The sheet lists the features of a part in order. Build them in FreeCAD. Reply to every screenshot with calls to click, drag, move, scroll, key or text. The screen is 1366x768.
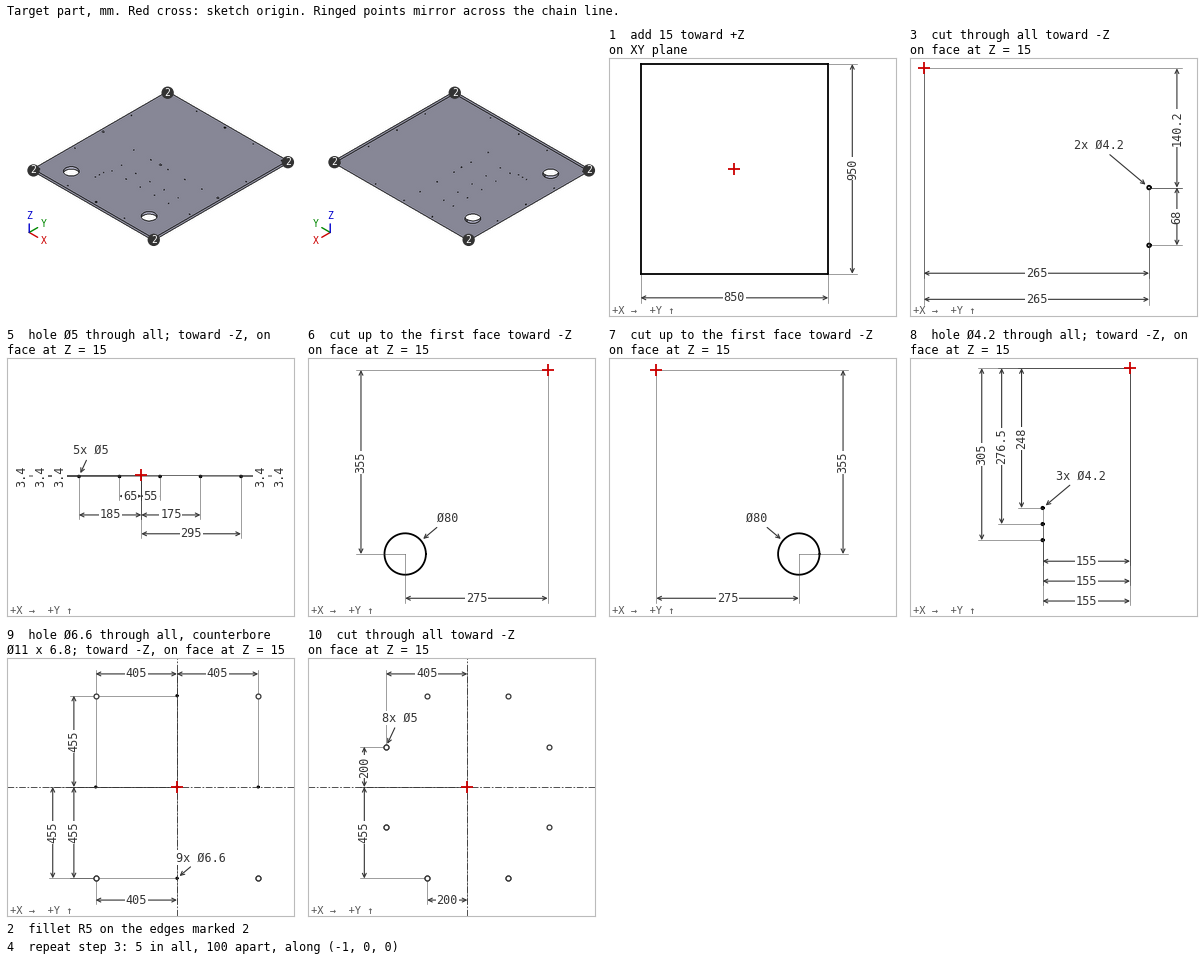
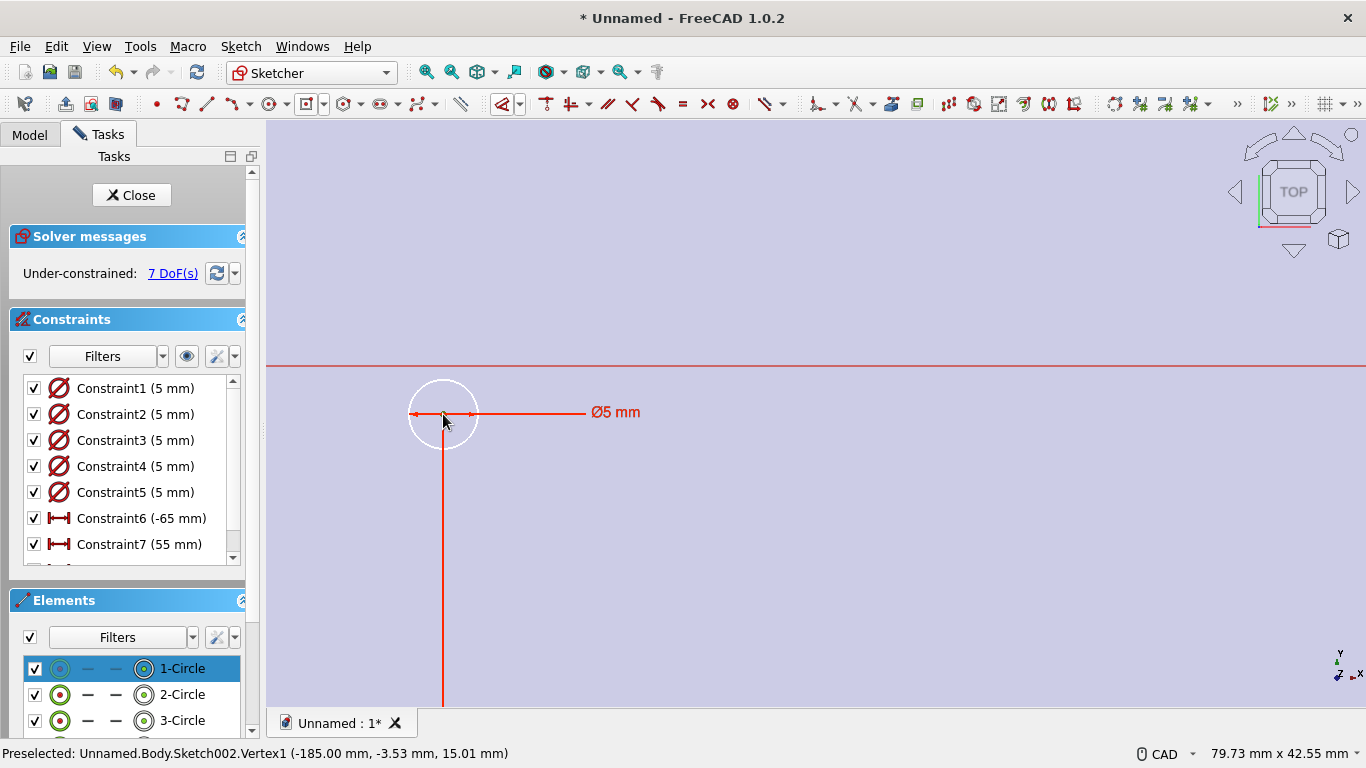
click(520, 104)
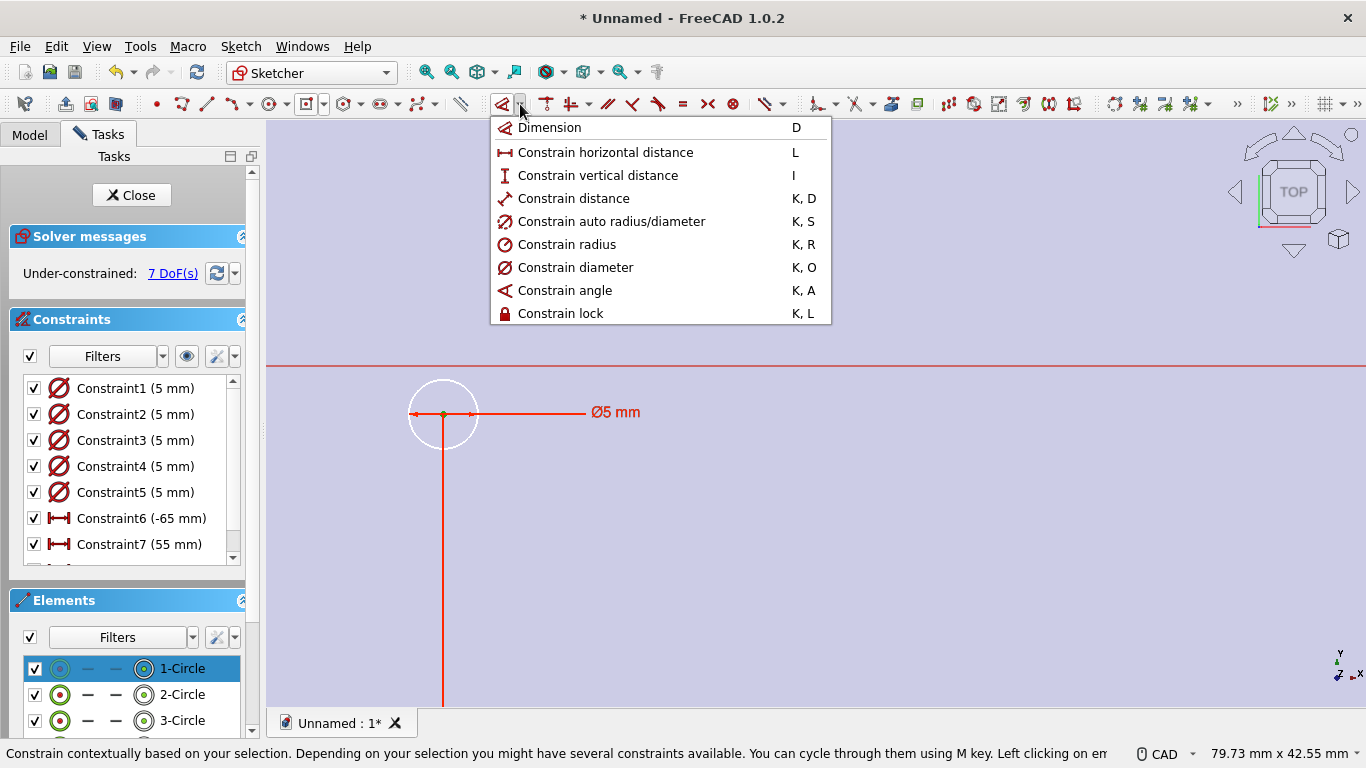
click(661, 176)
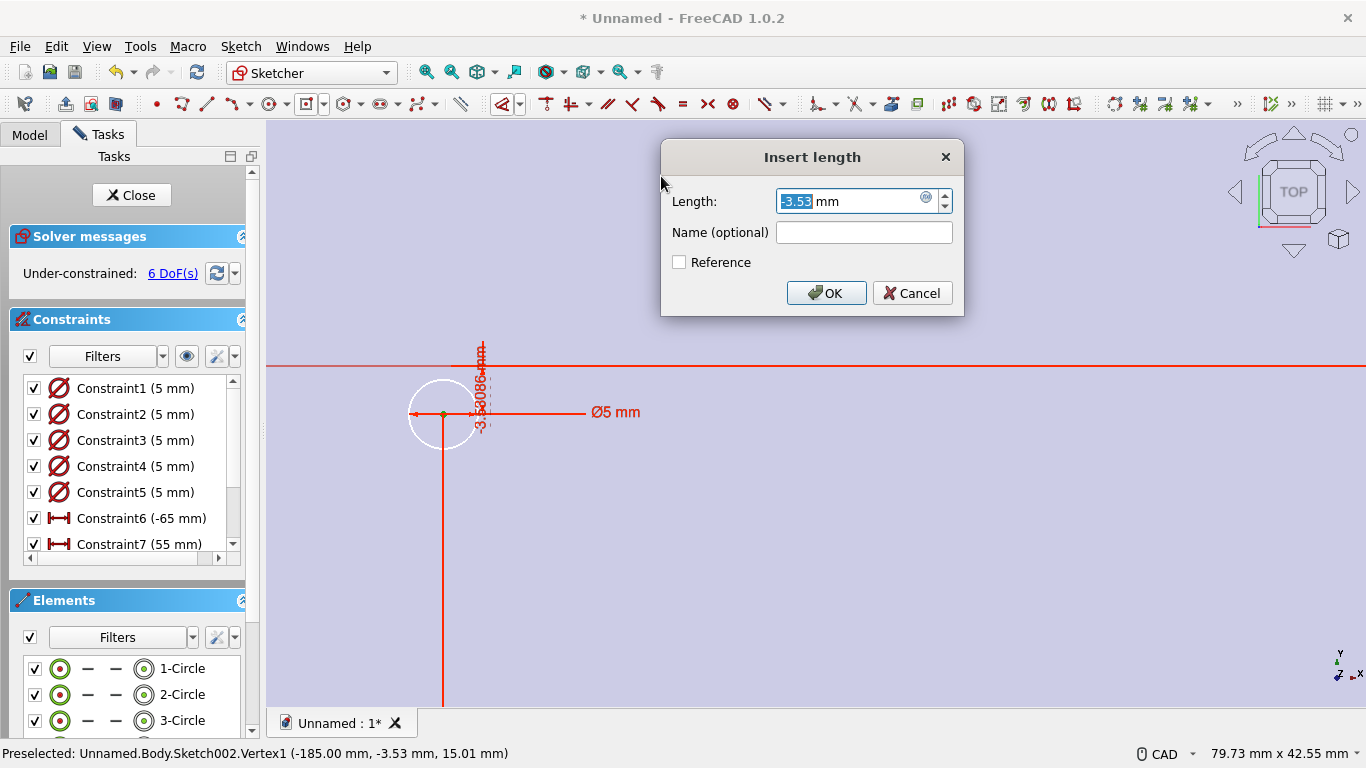
text(-3.4)
key(Return)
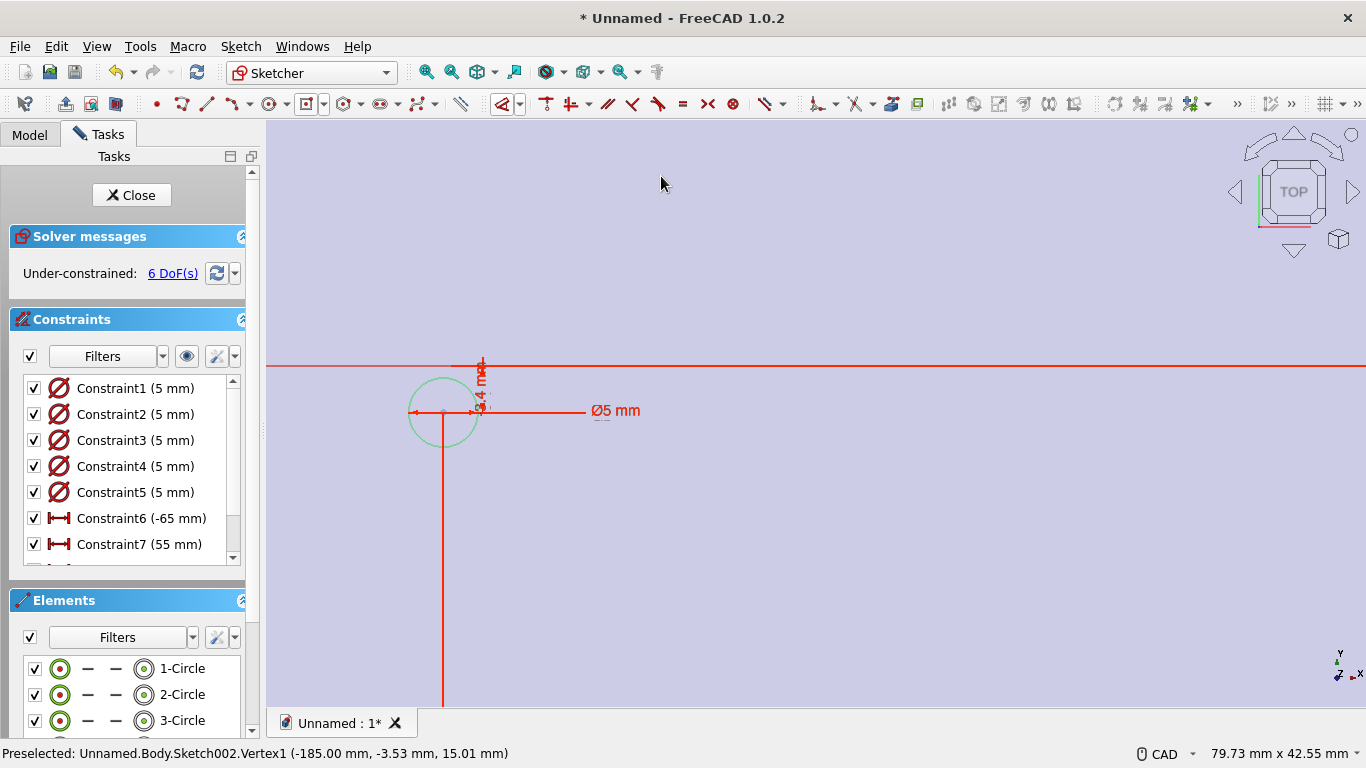
scroll(447, 414, down, 12)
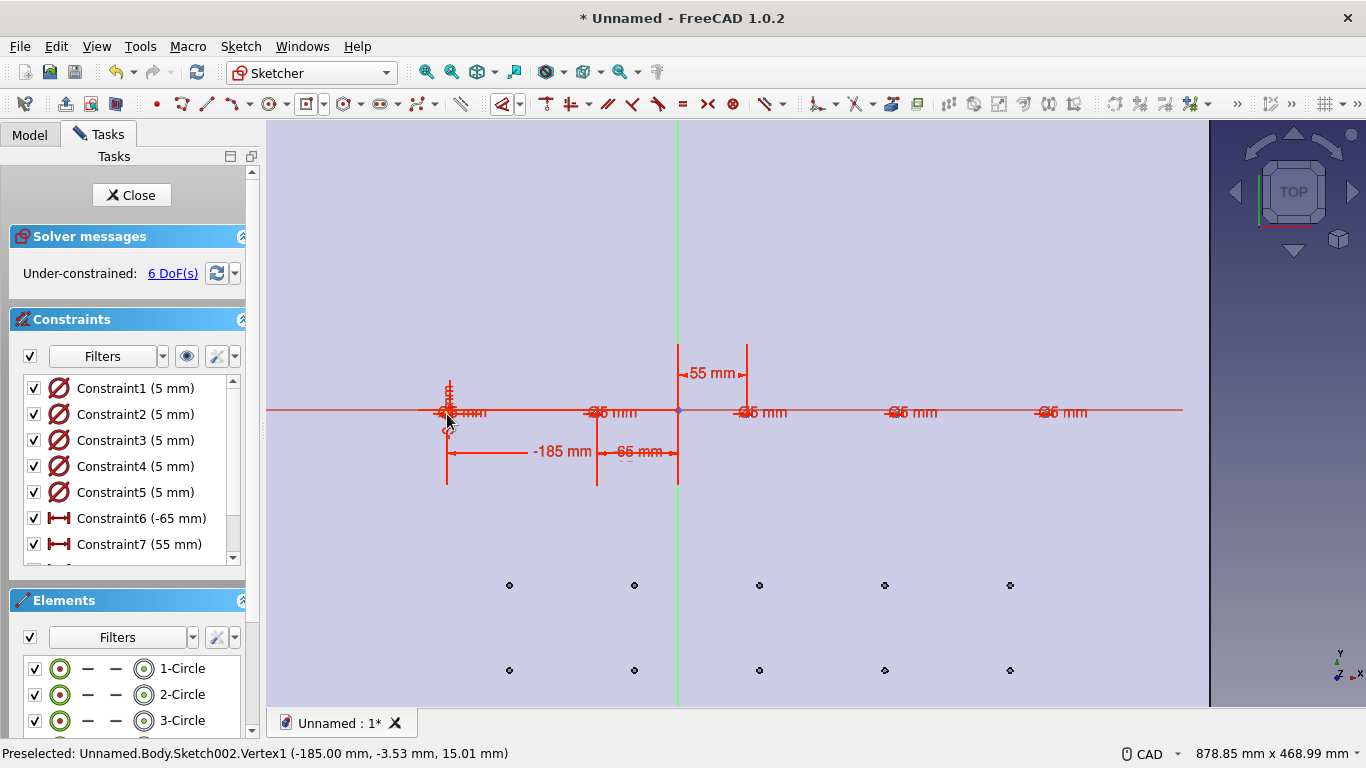
scroll(597, 414, up, 12)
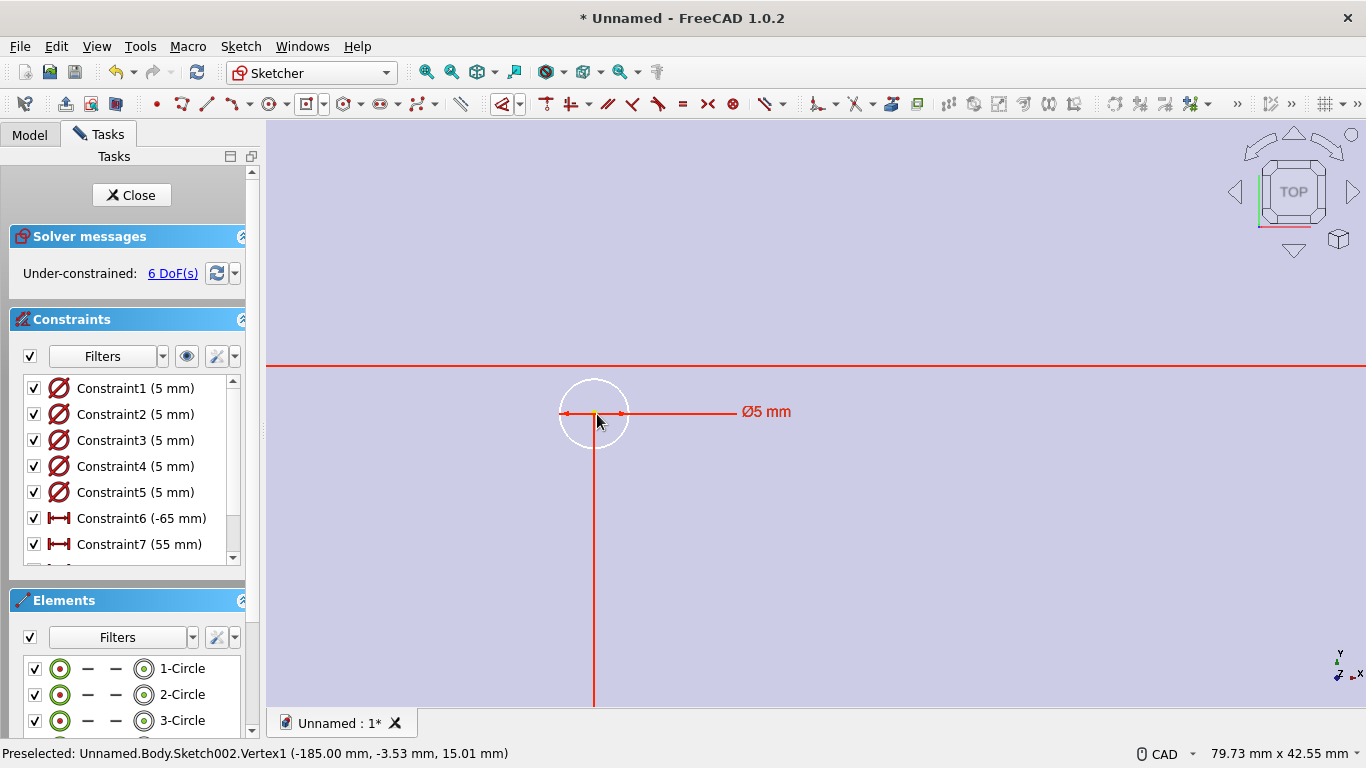
click(594, 414)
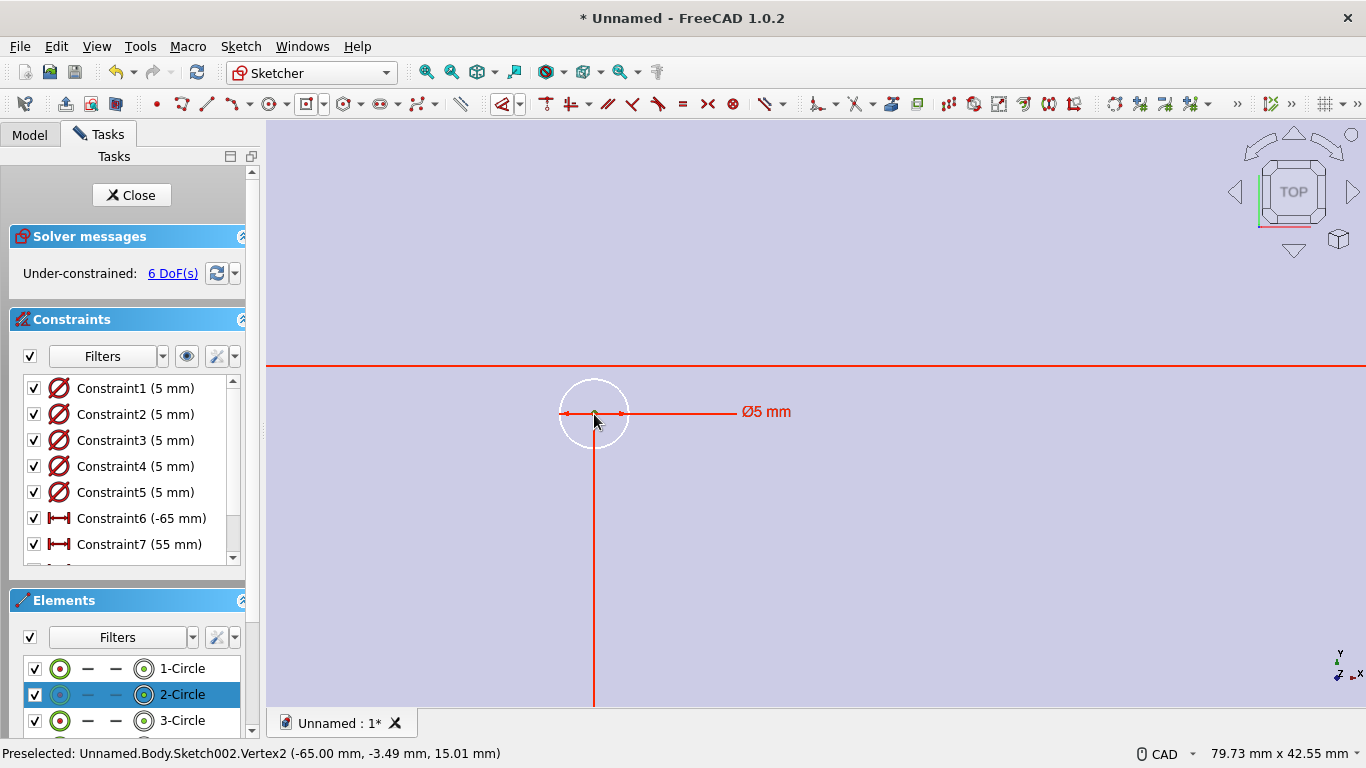
click(520, 104)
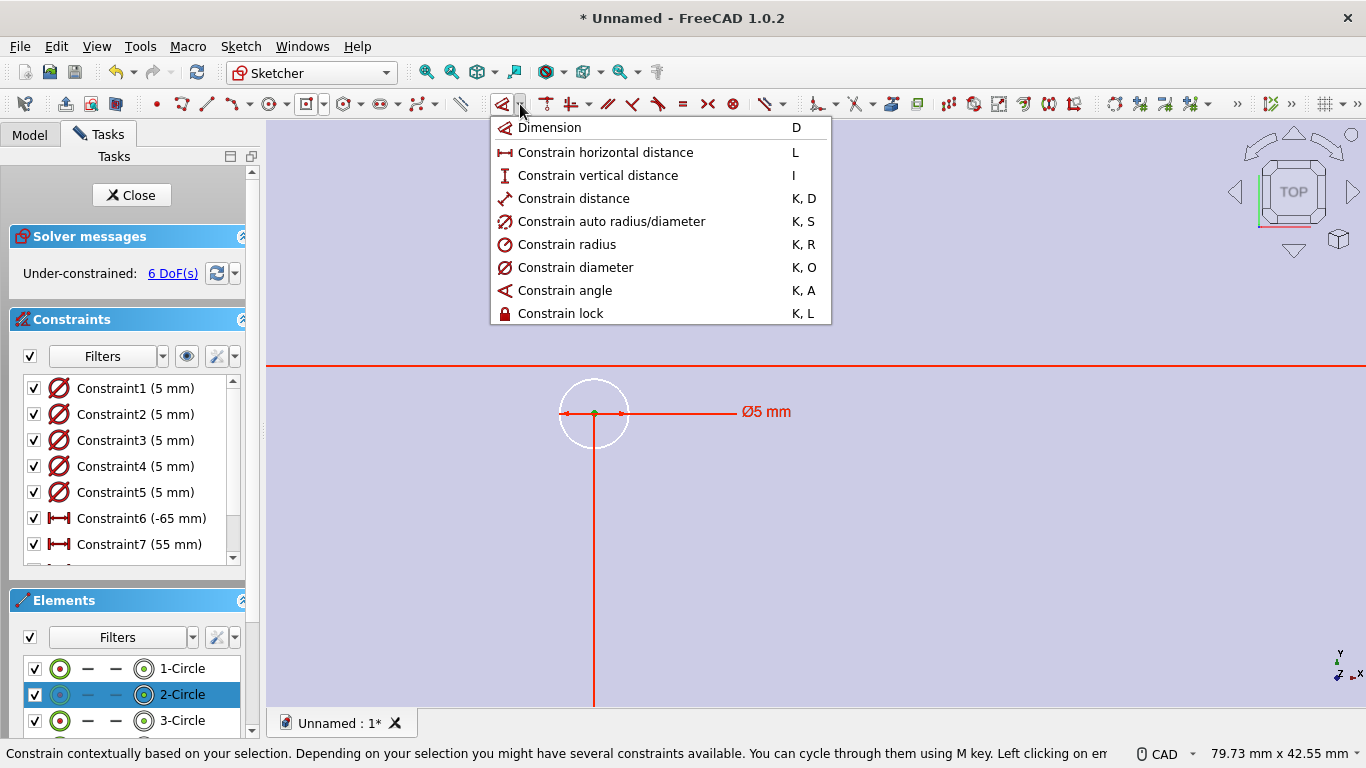
click(661, 176)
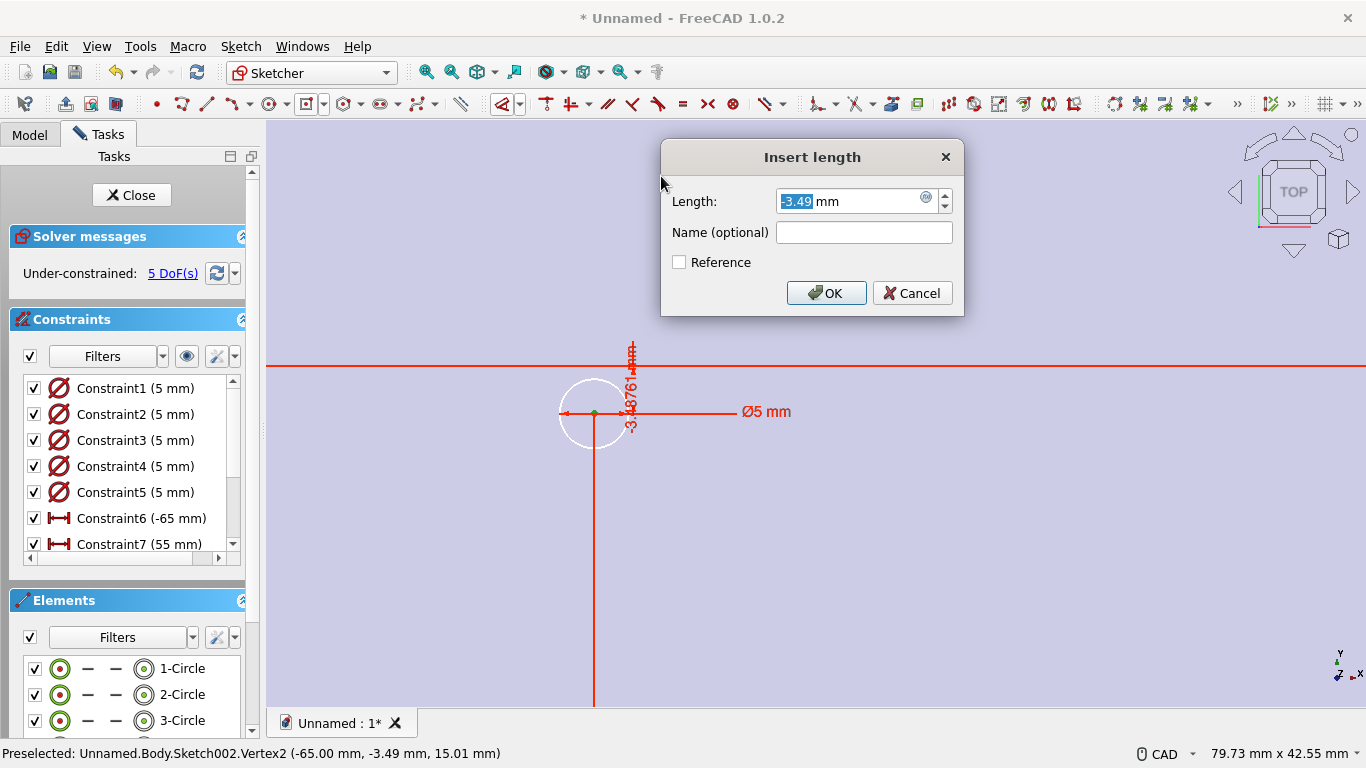
text(-3.4)
key(Return)